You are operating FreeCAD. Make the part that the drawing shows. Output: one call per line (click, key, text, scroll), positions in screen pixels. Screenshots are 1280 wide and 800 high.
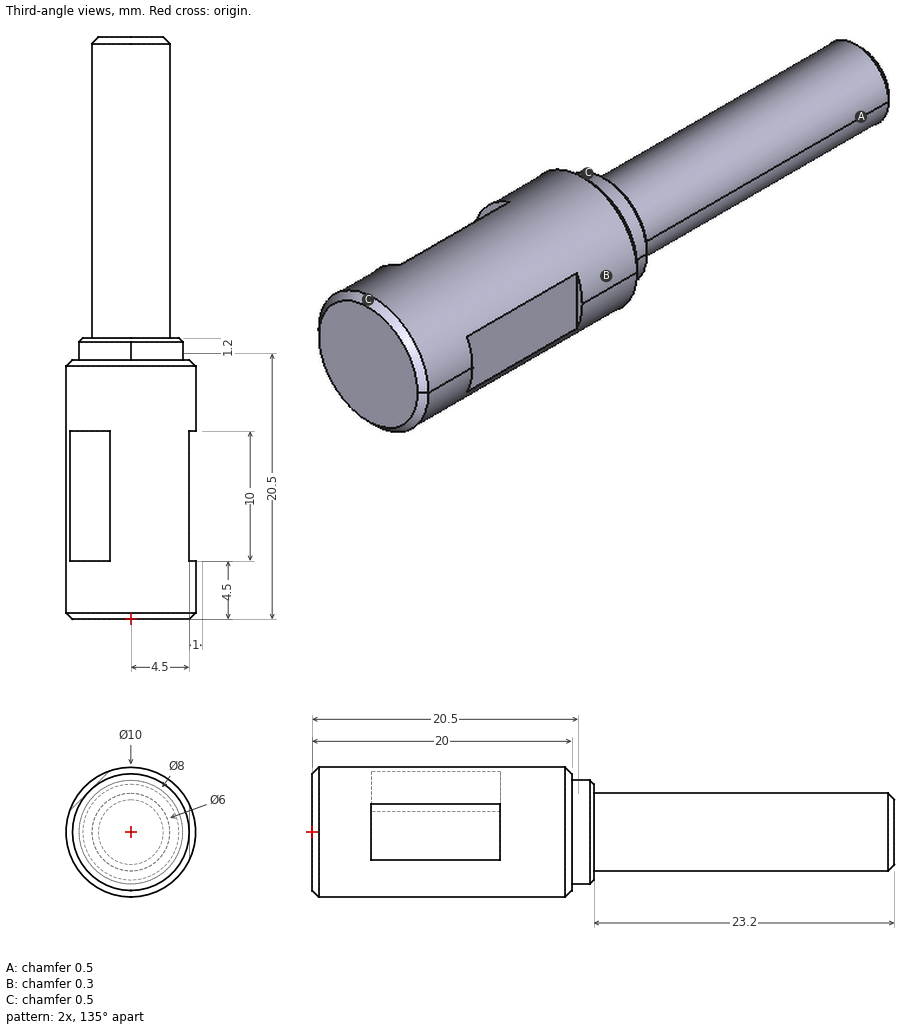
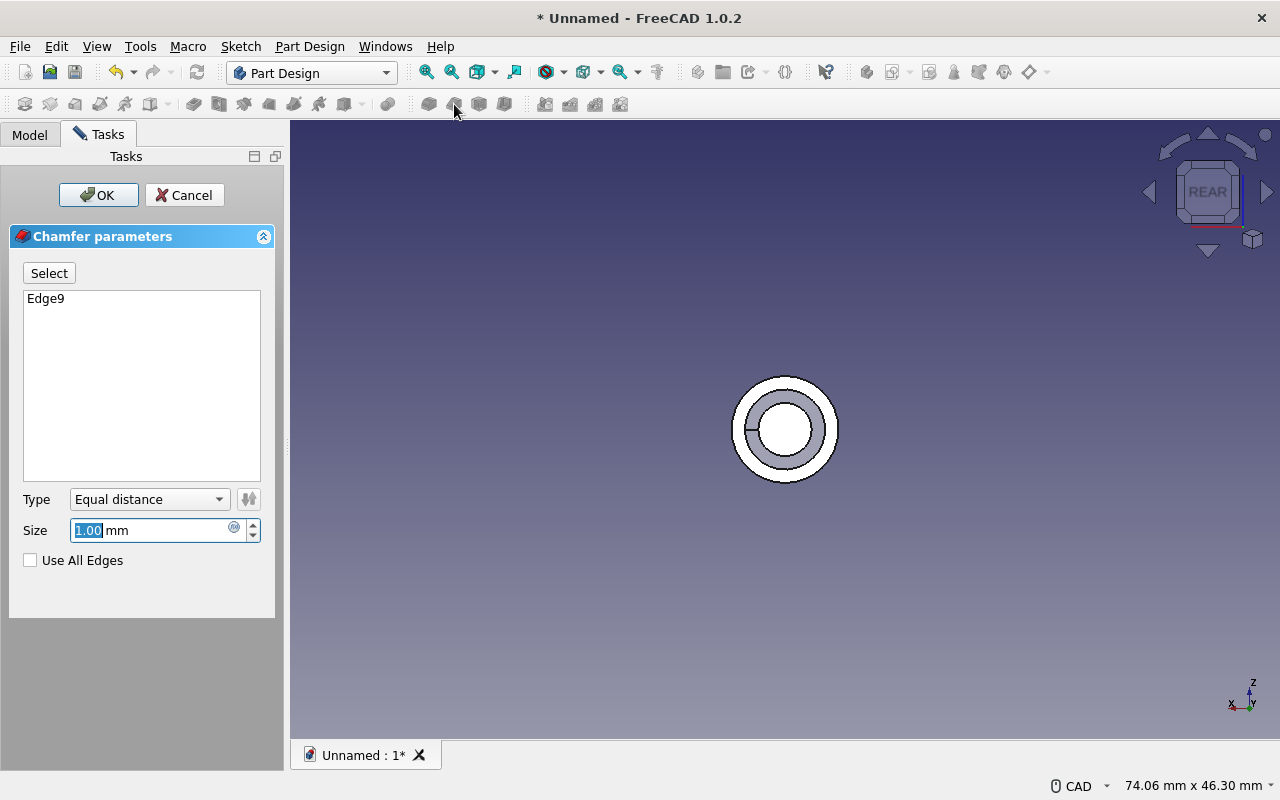
text(0.5)
key(Tab)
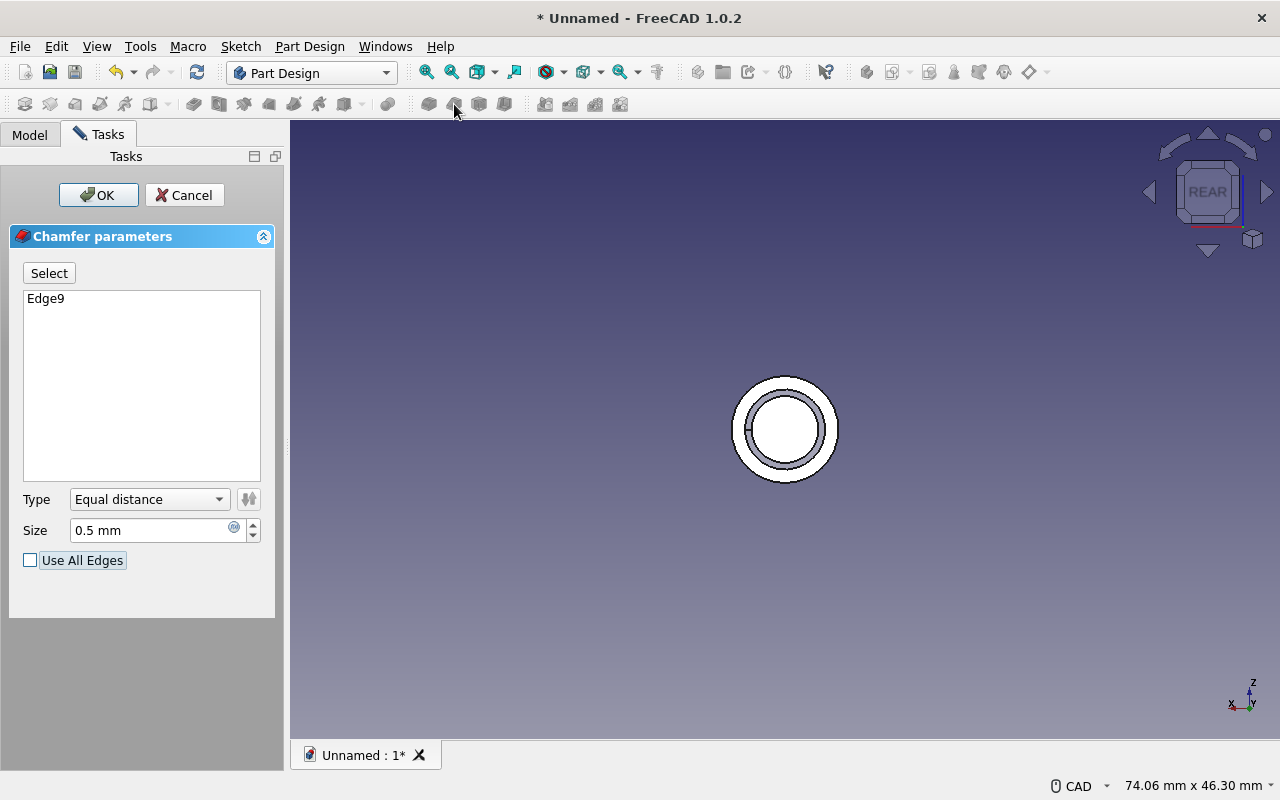
click(99, 195)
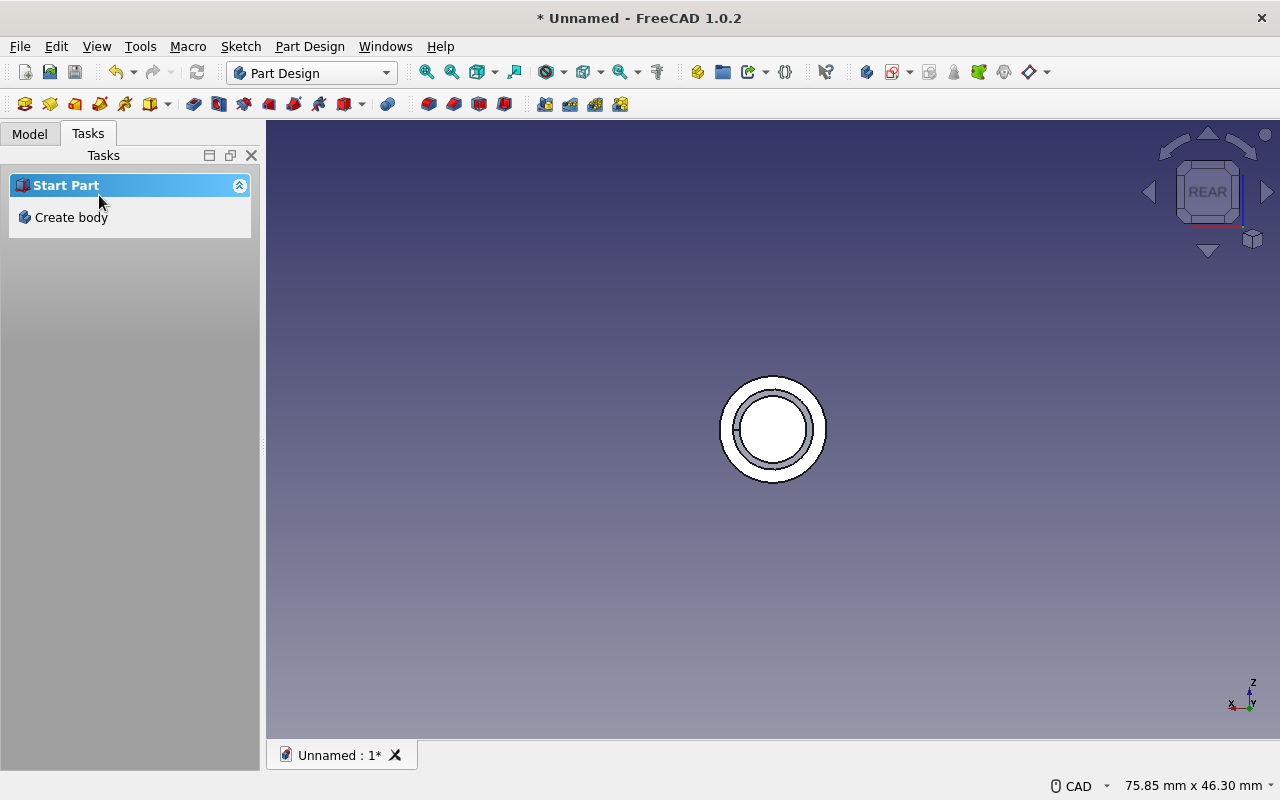
click(427, 72)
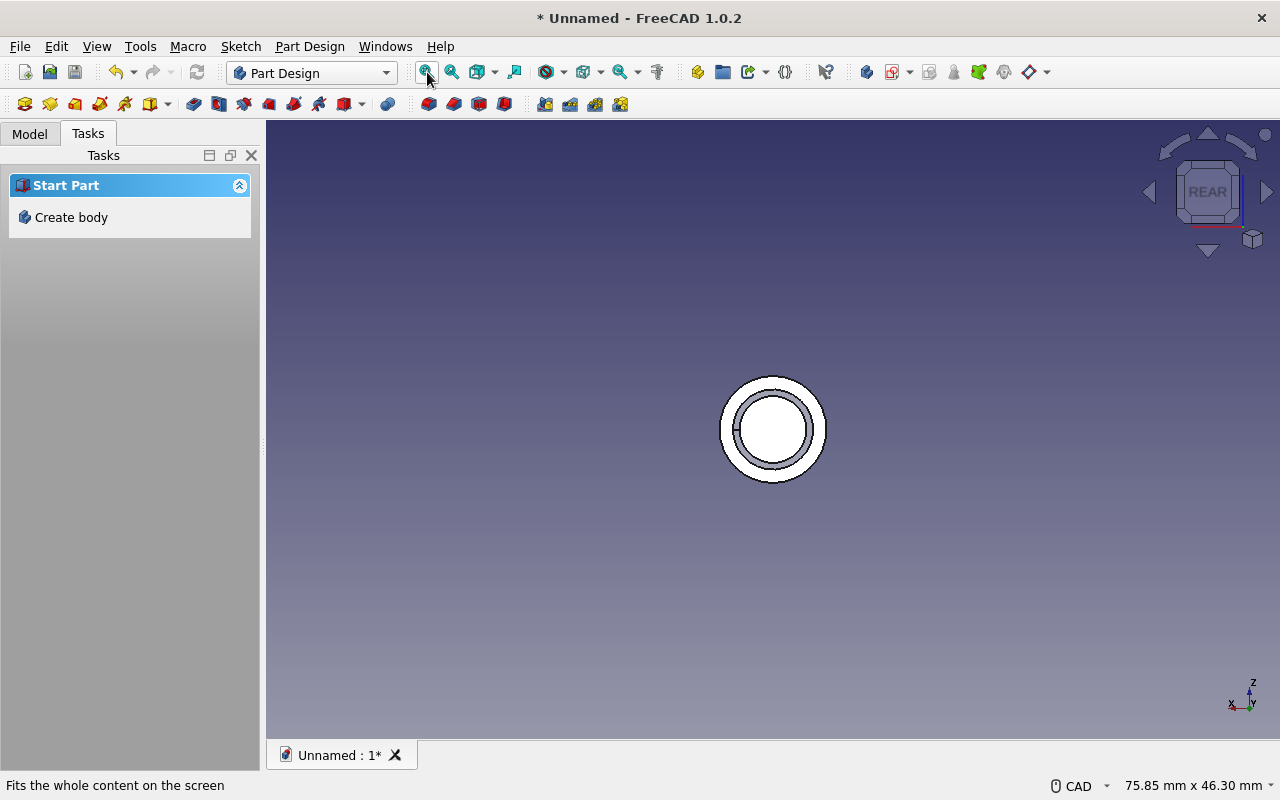
click(892, 72)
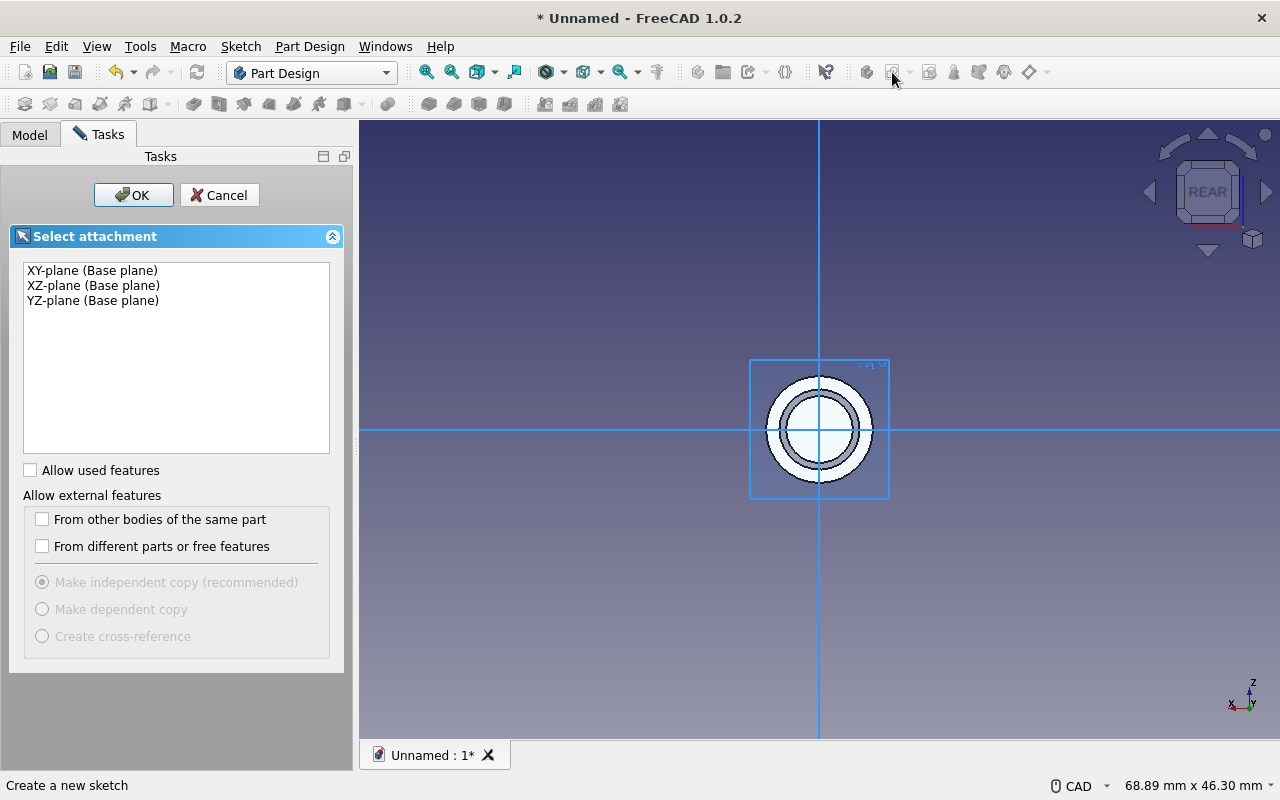
click(84, 286)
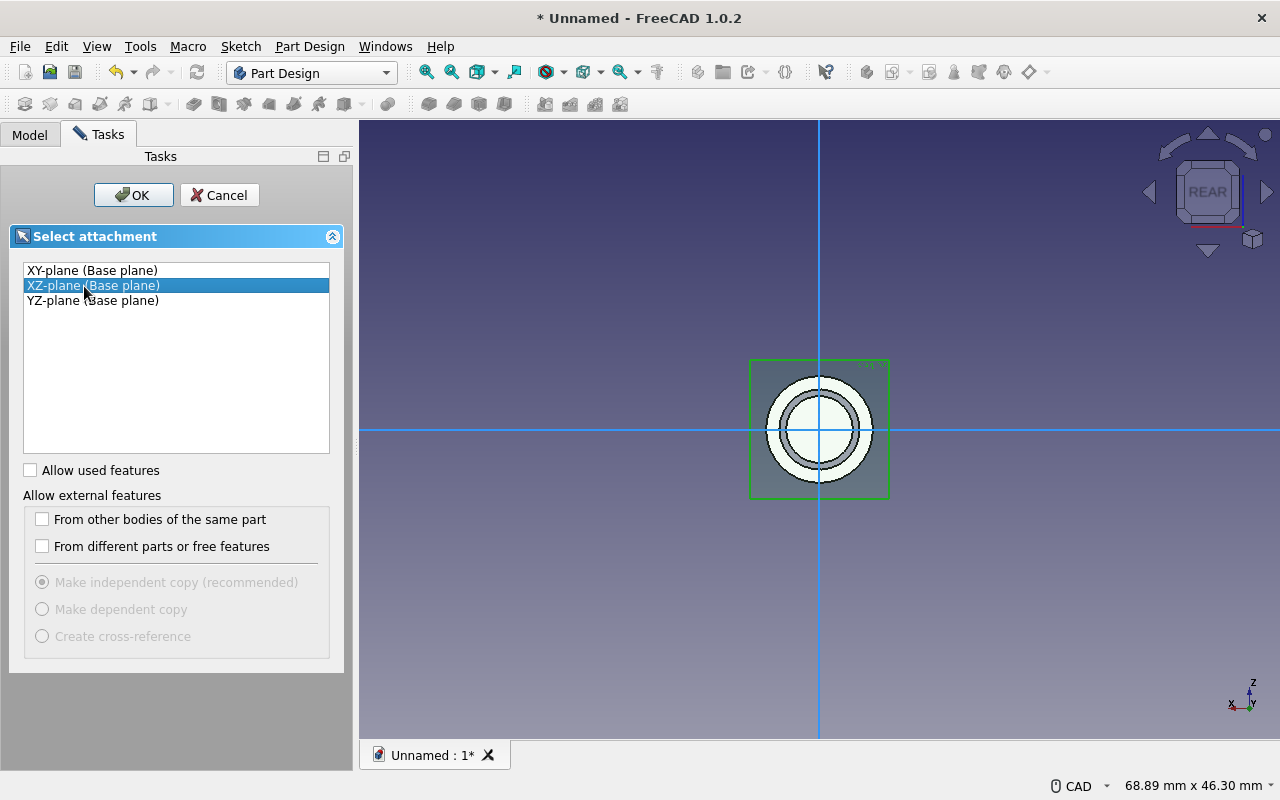
click(134, 195)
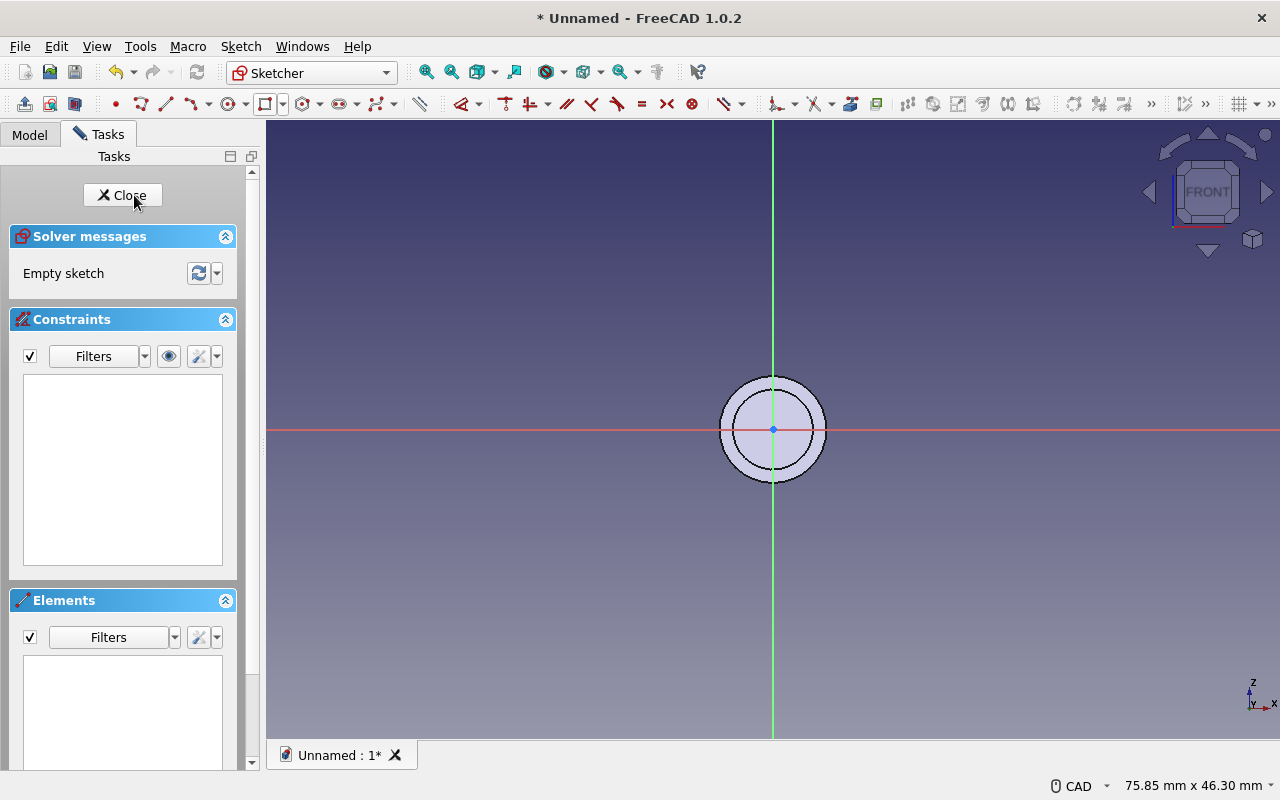
scroll(795, 430, up, 7)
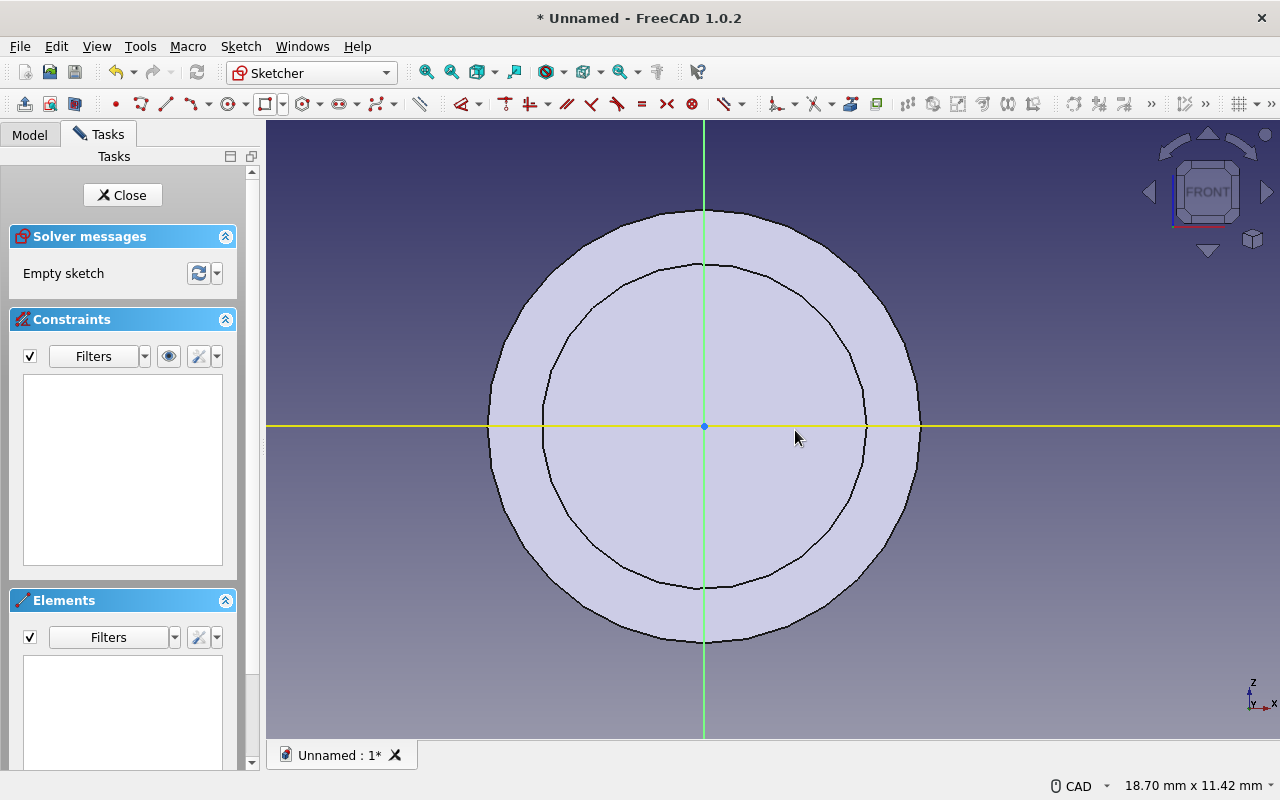
click(228, 104)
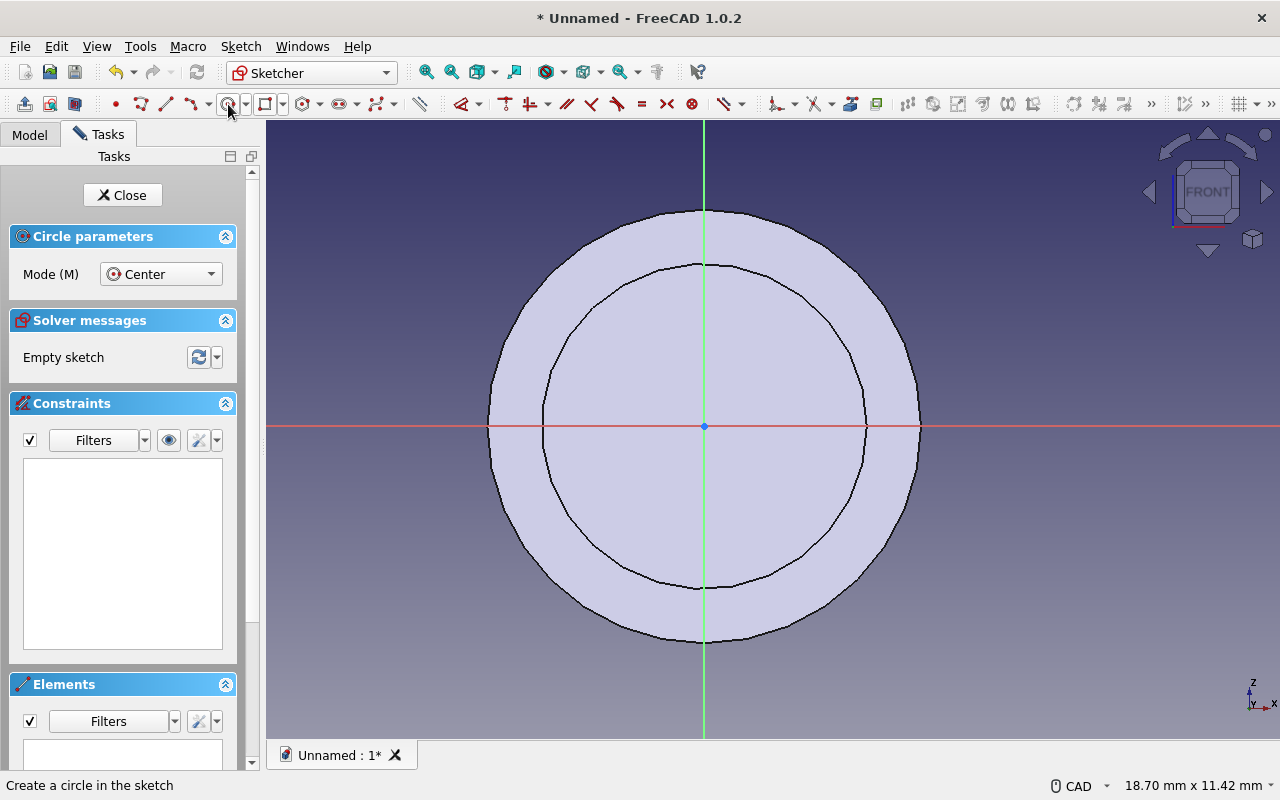
click(704, 426)
move(858, 273)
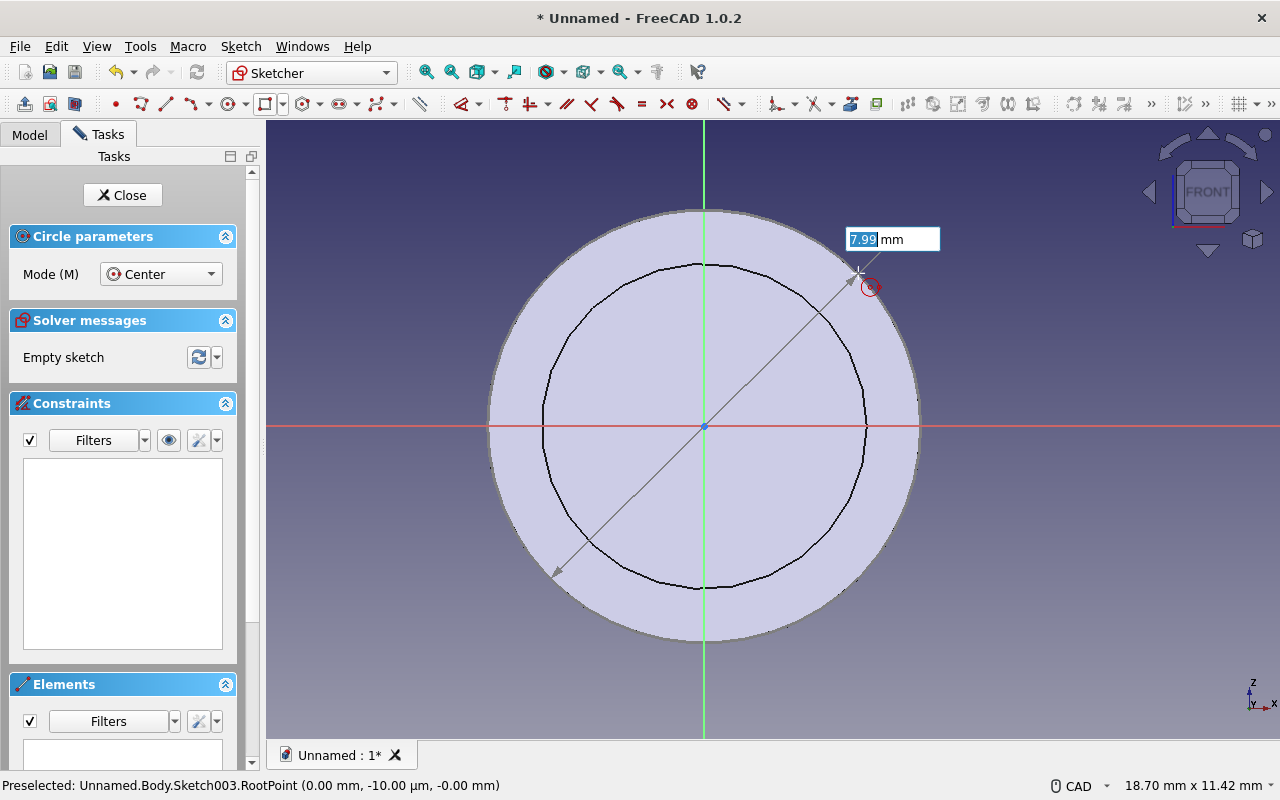
text(8)
key(Return)
key(Escape)